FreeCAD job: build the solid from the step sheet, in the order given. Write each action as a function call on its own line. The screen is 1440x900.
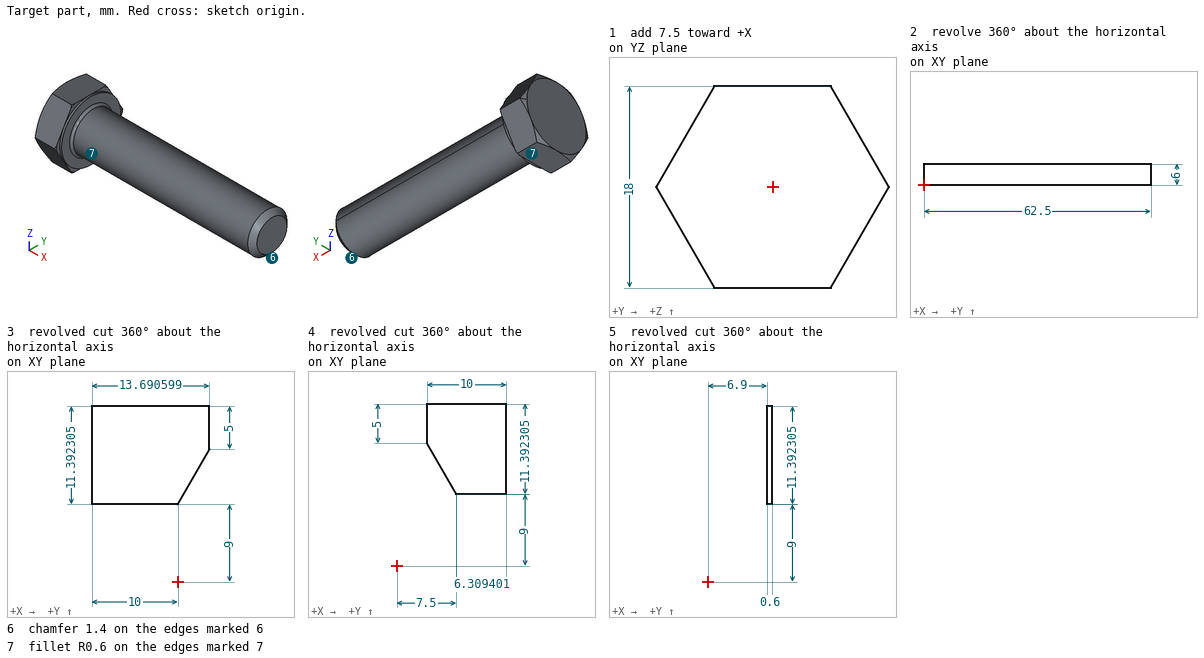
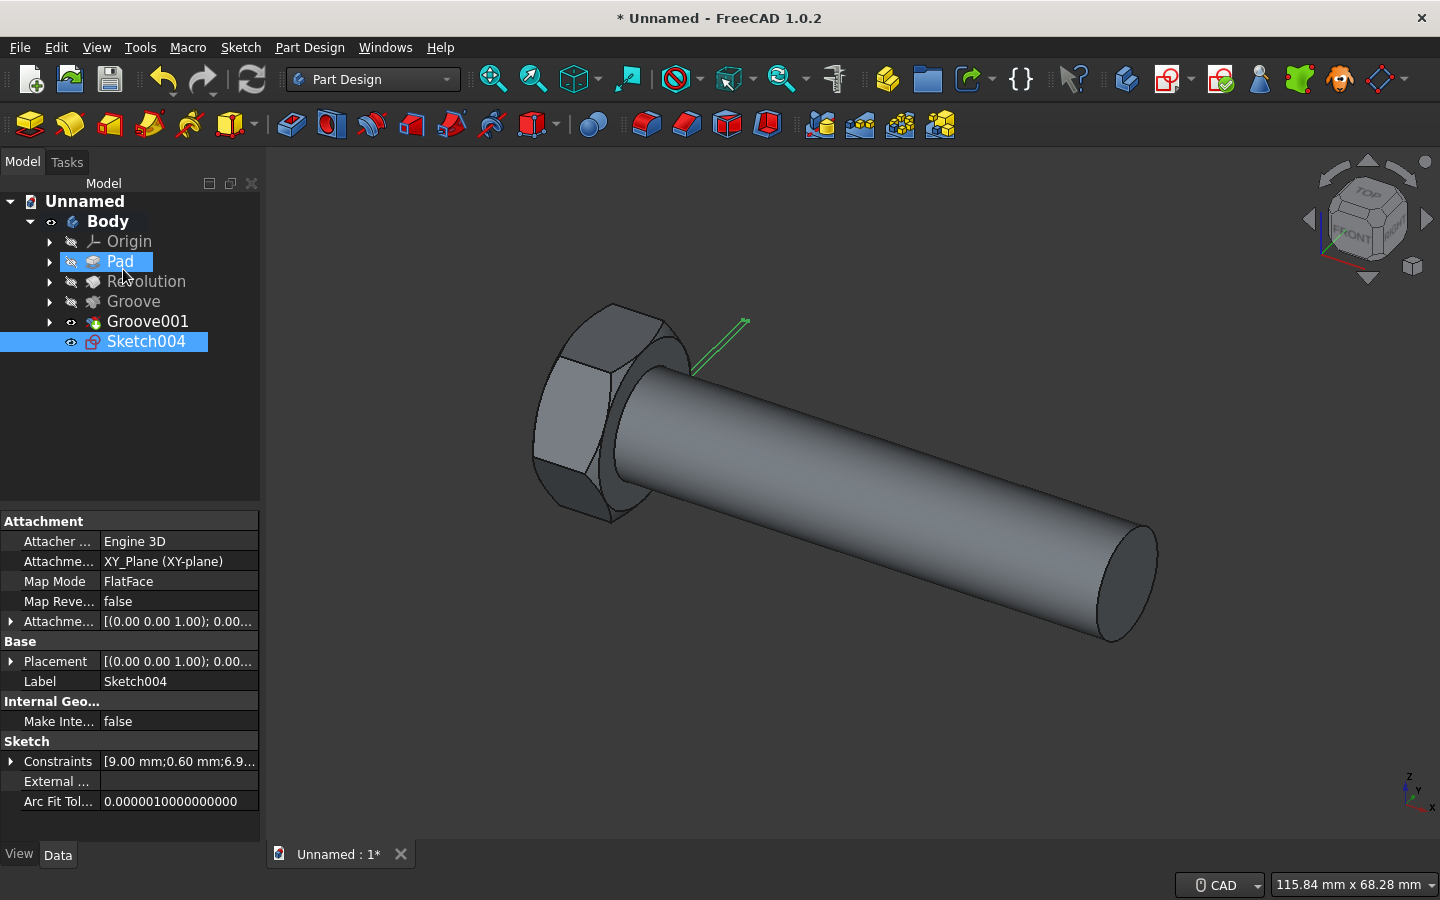
click(372, 124)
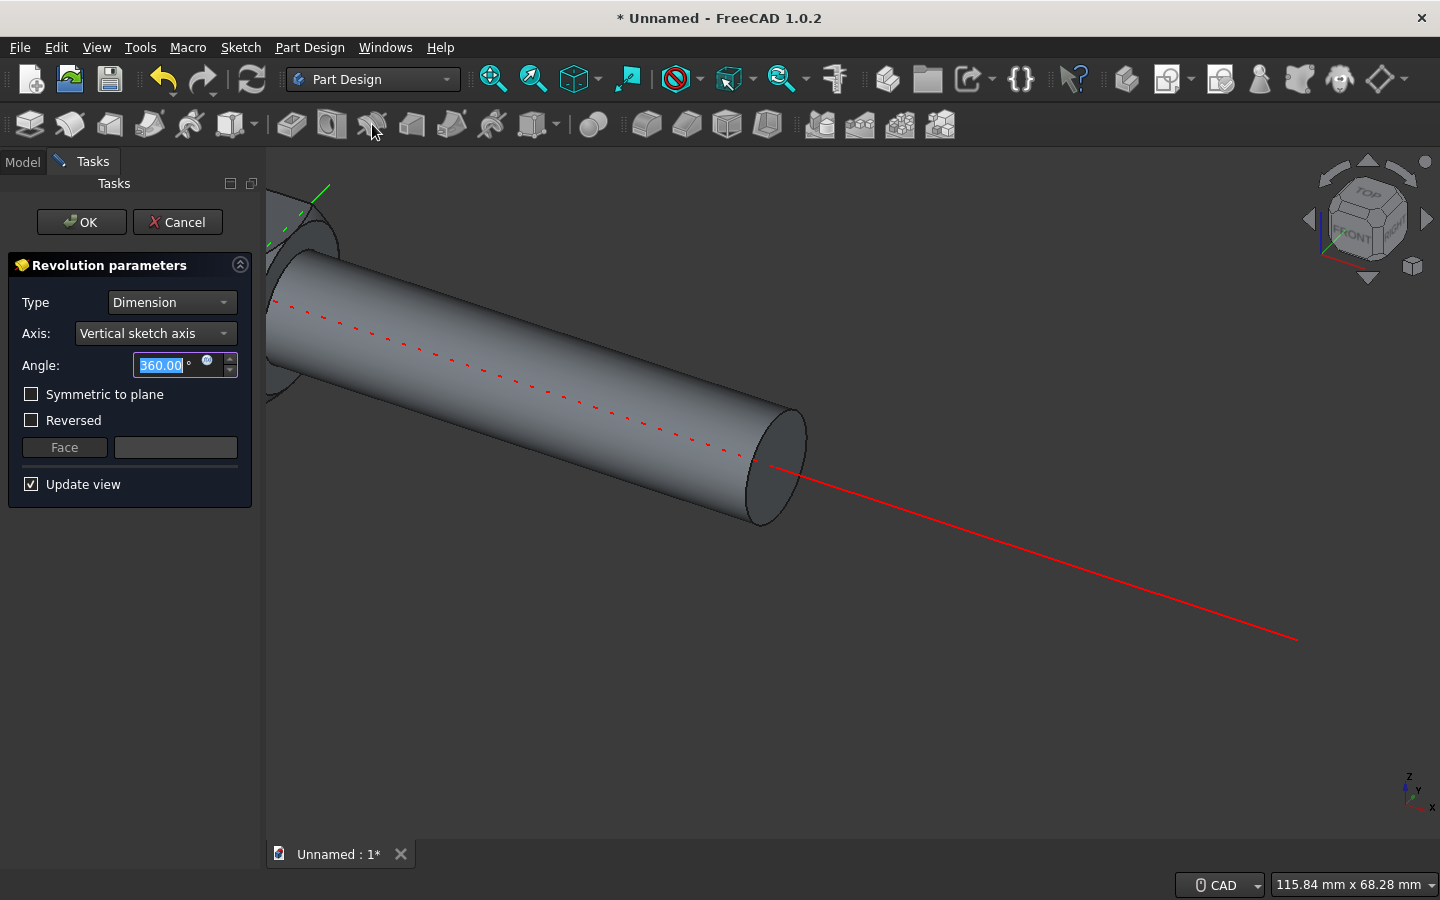
click(156, 334)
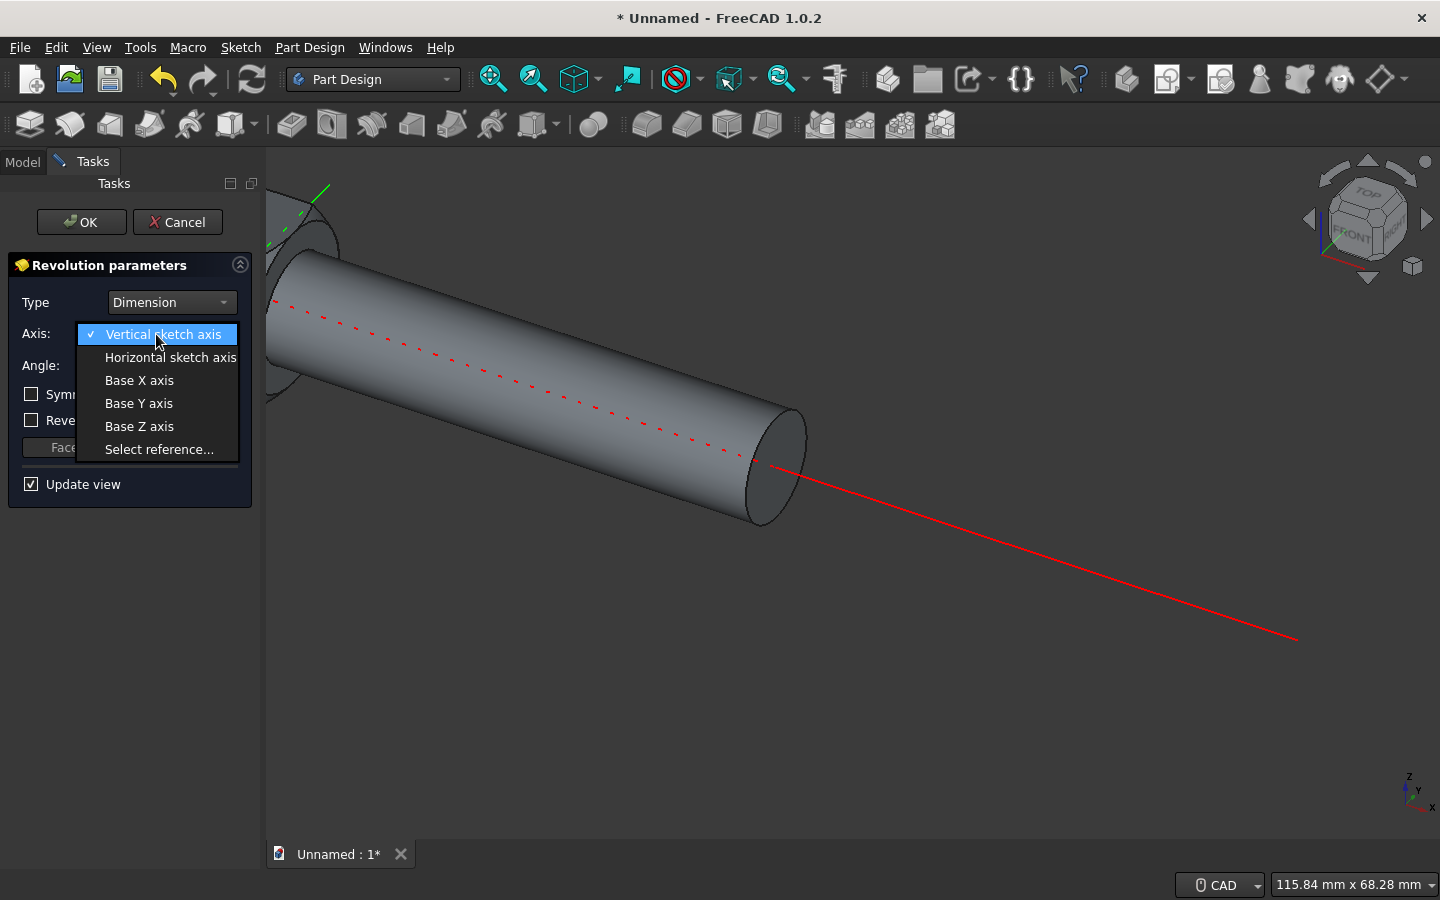
click(156, 358)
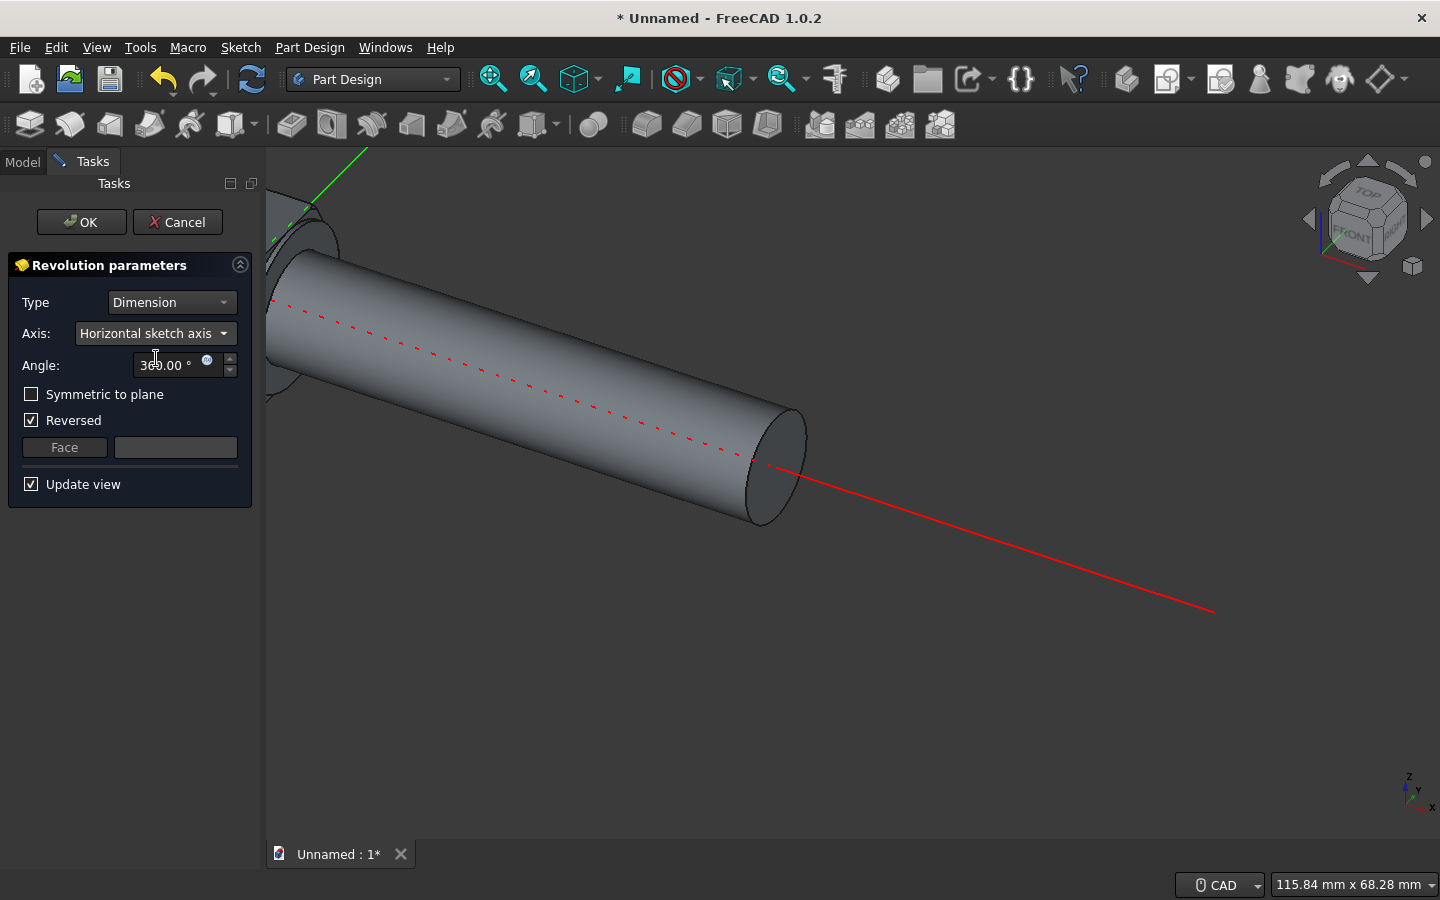
click(82, 222)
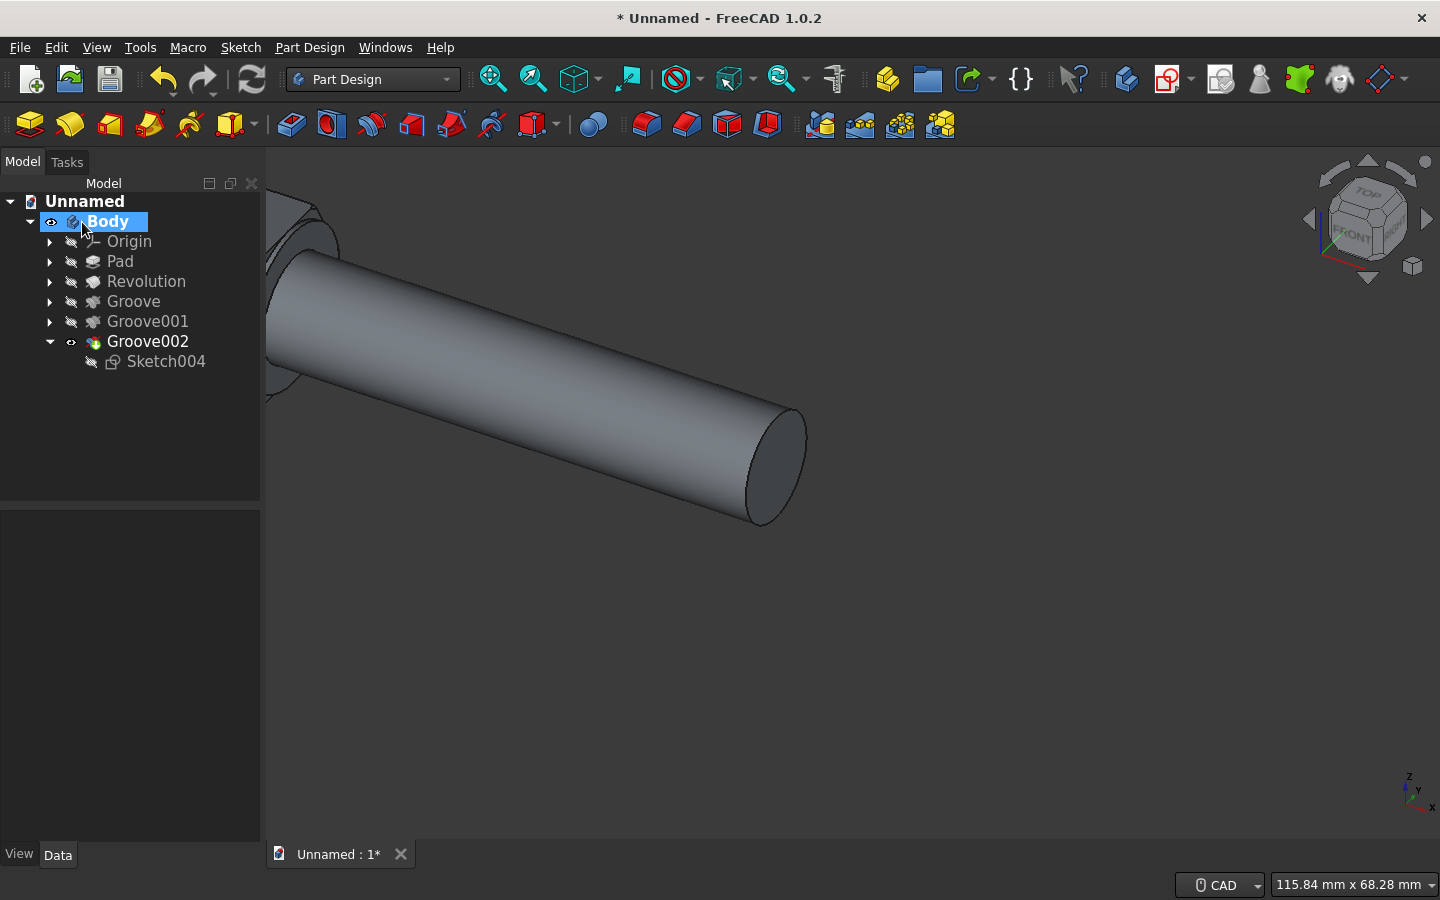
click(494, 80)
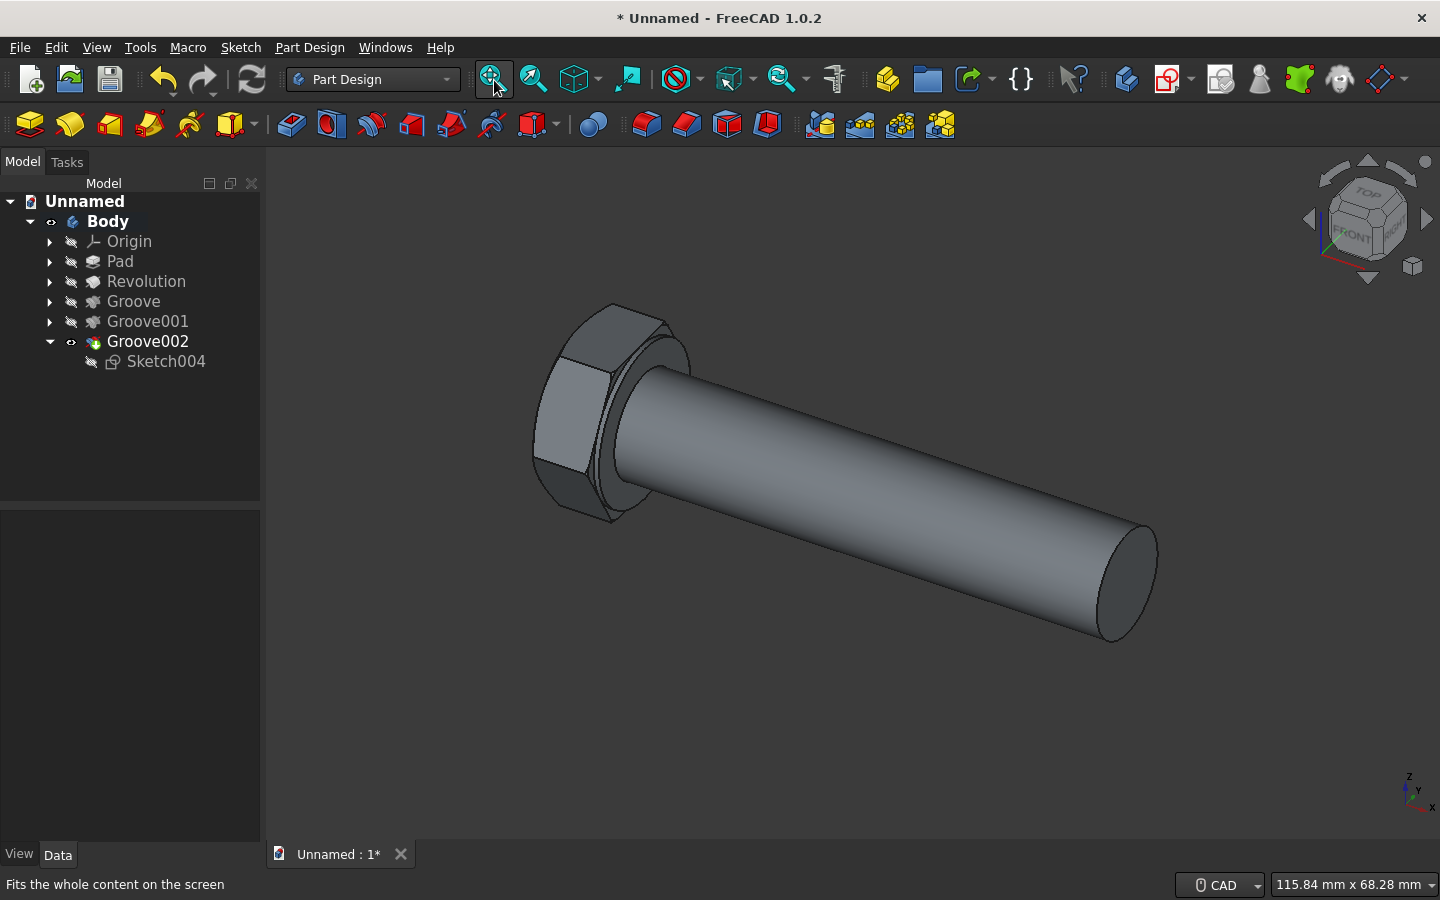
click(1097, 613)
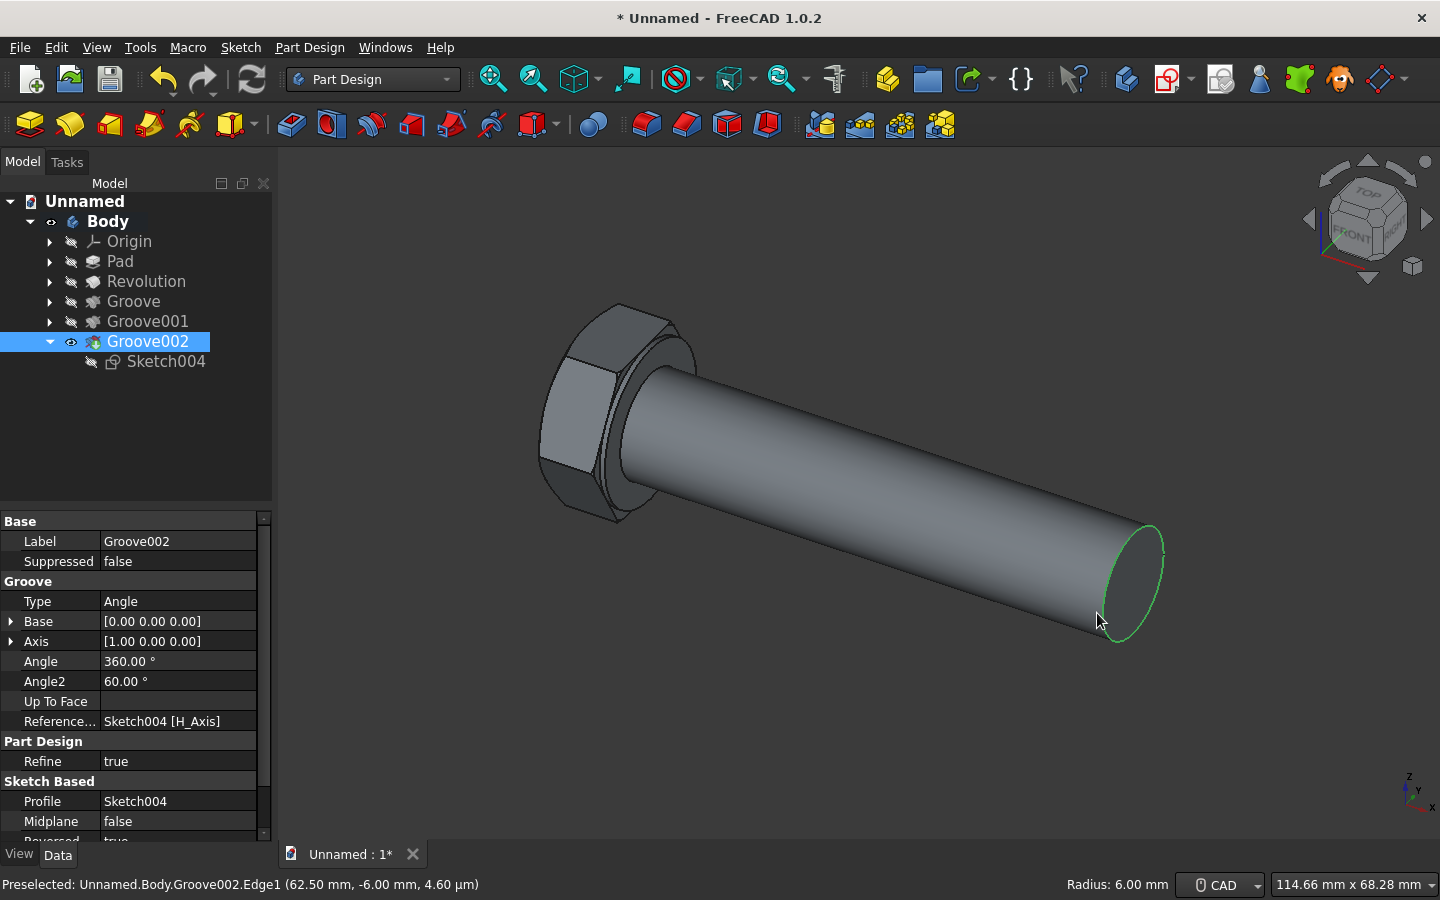
click(688, 124)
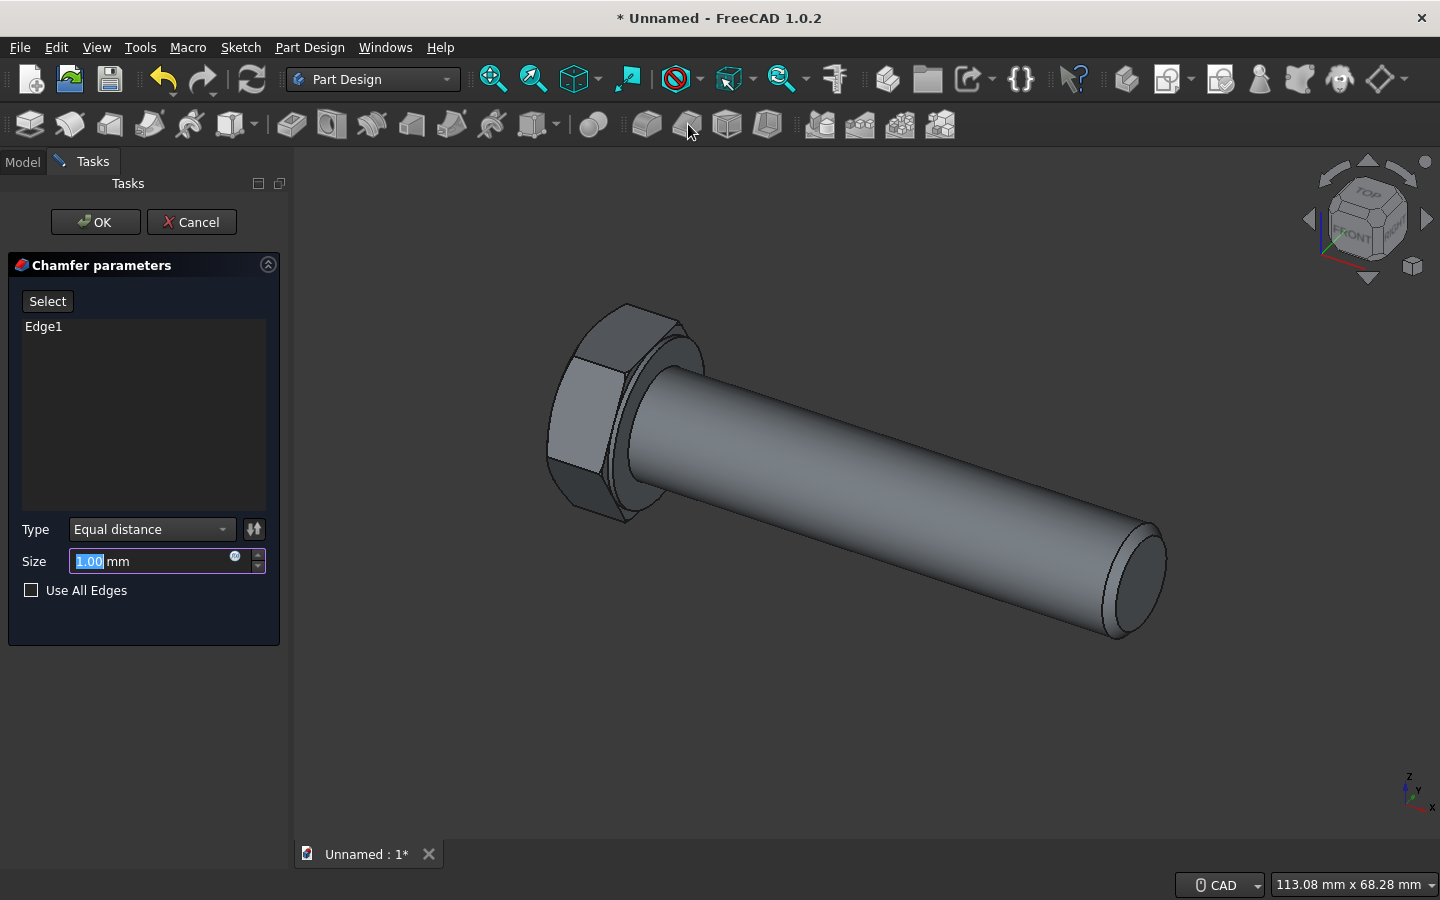
text(1.4)
key(Tab)